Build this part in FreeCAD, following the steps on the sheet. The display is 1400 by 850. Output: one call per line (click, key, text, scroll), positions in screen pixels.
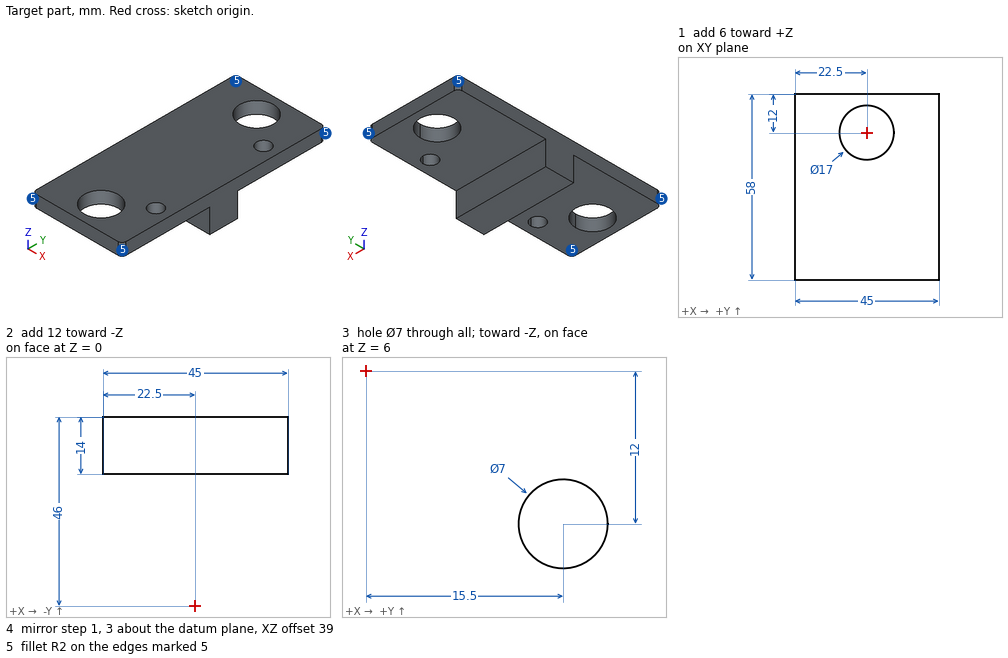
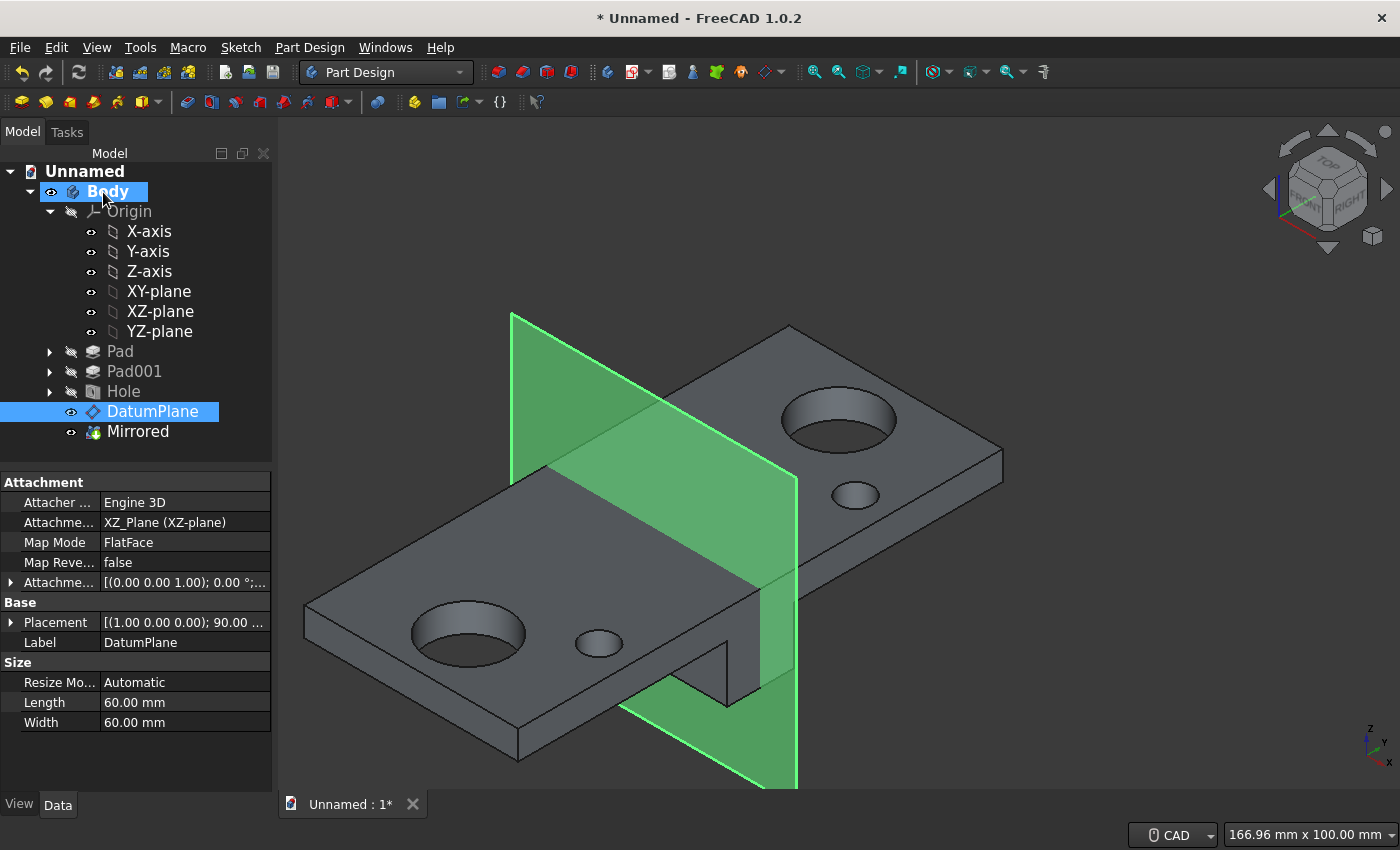
click(116, 412)
key(space)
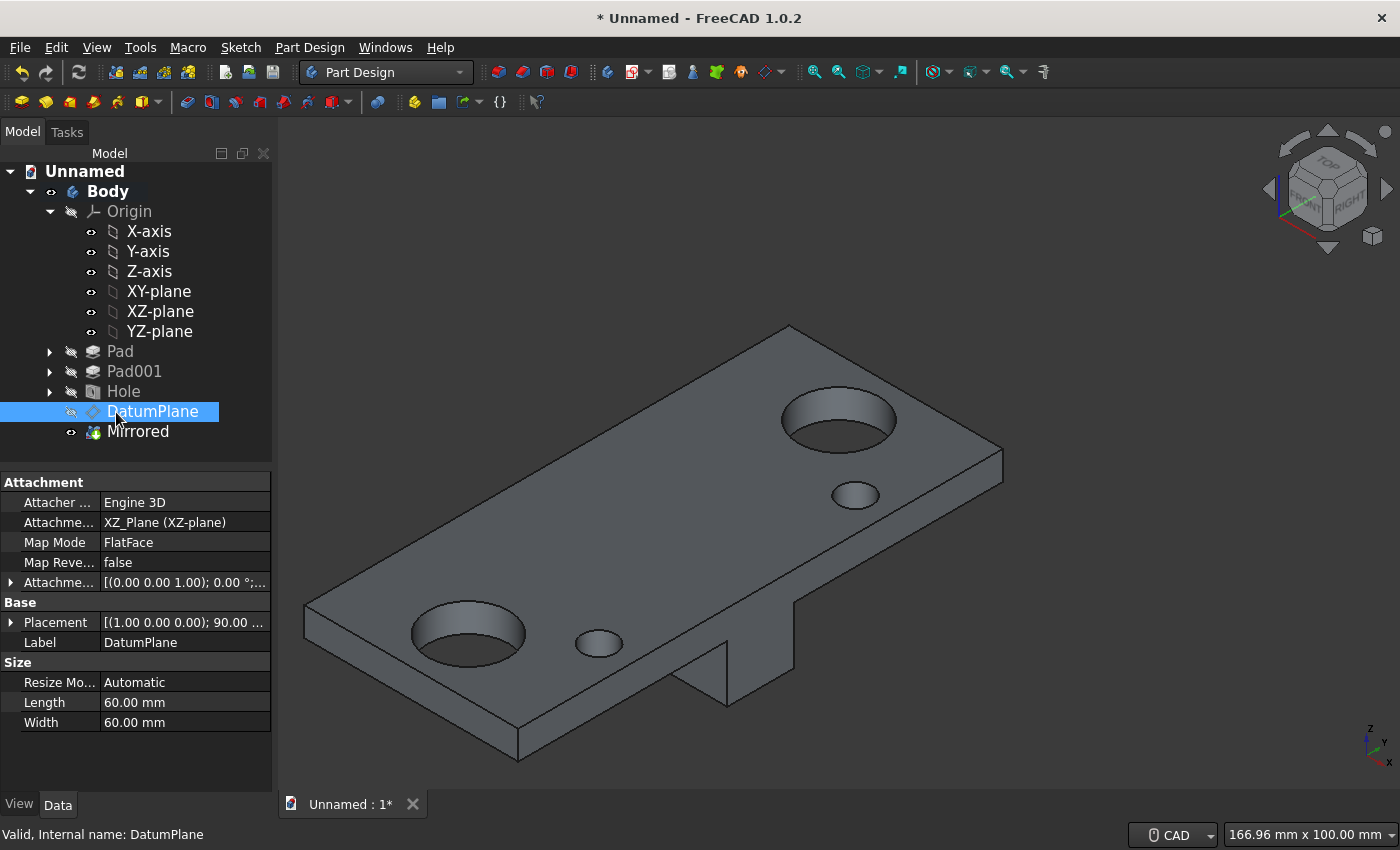
click(816, 72)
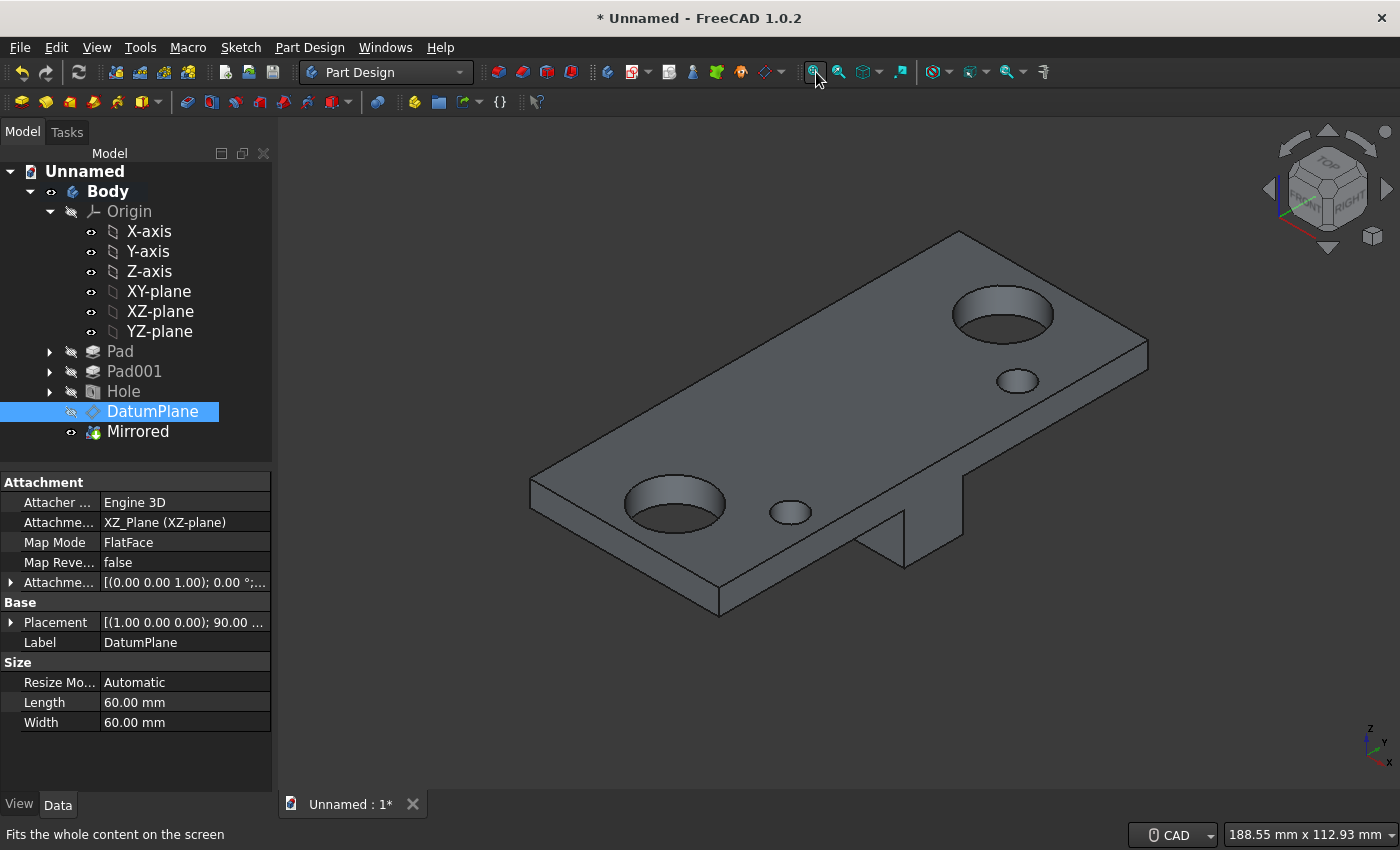
click(719, 601)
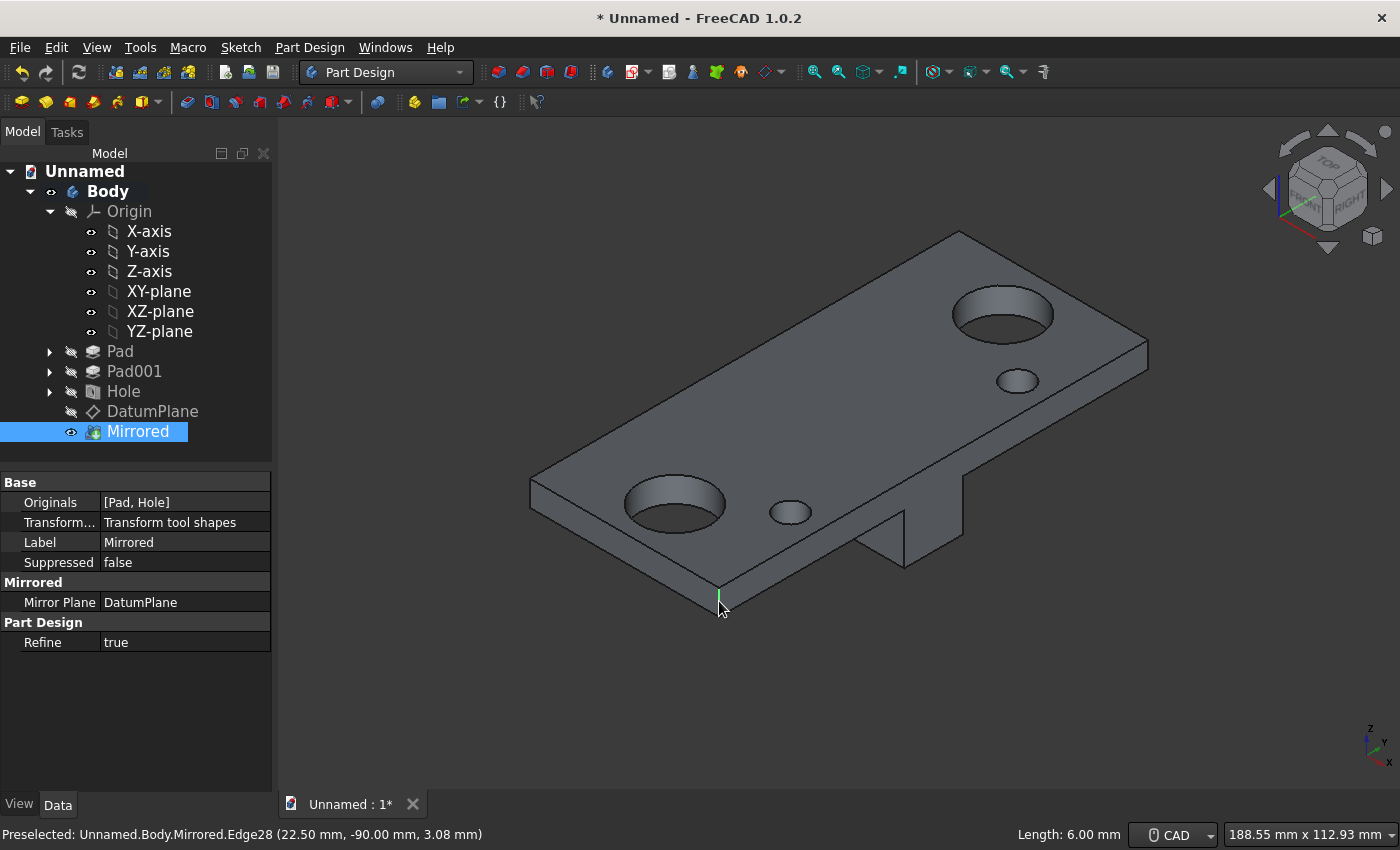
key(2)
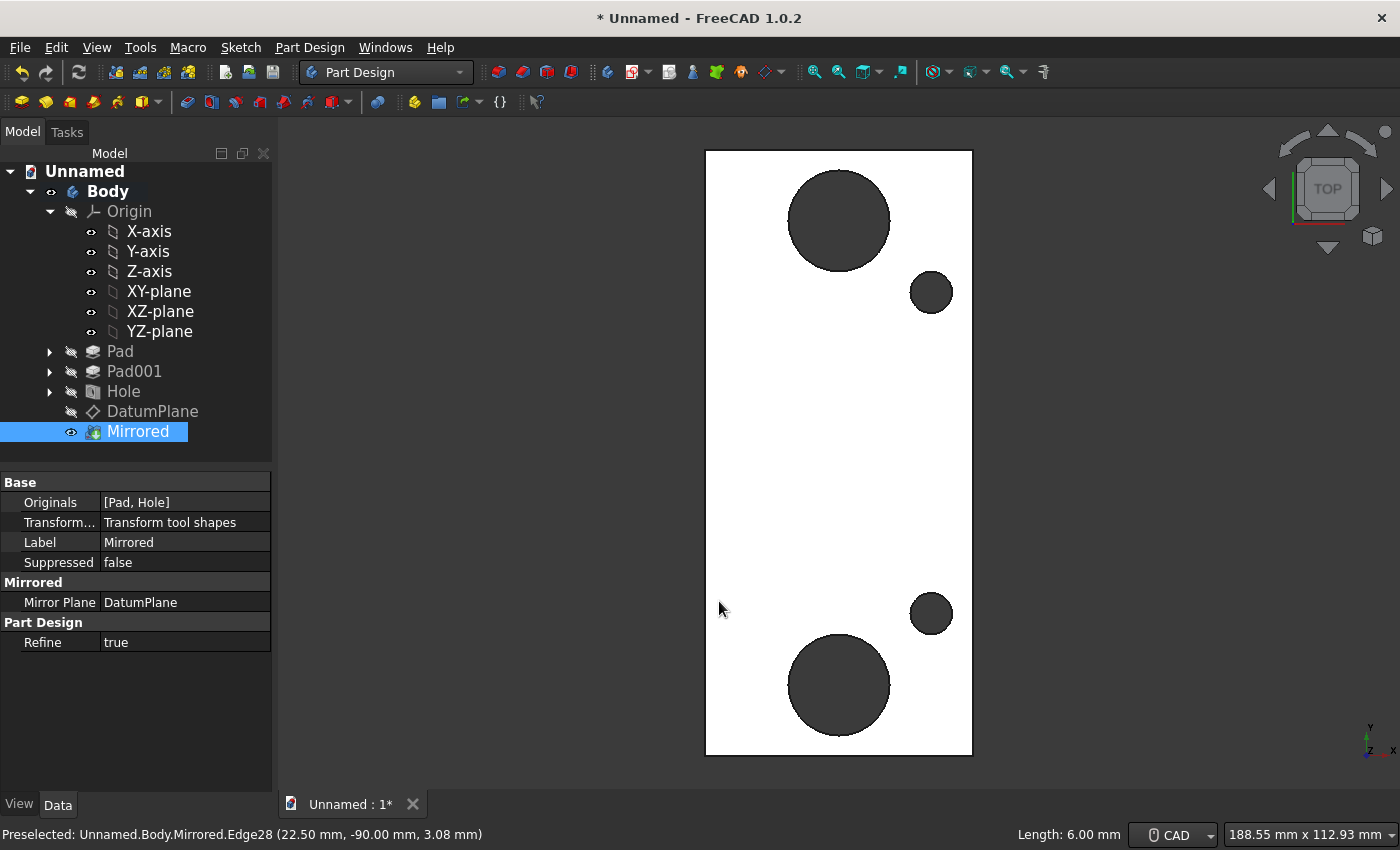
key(0)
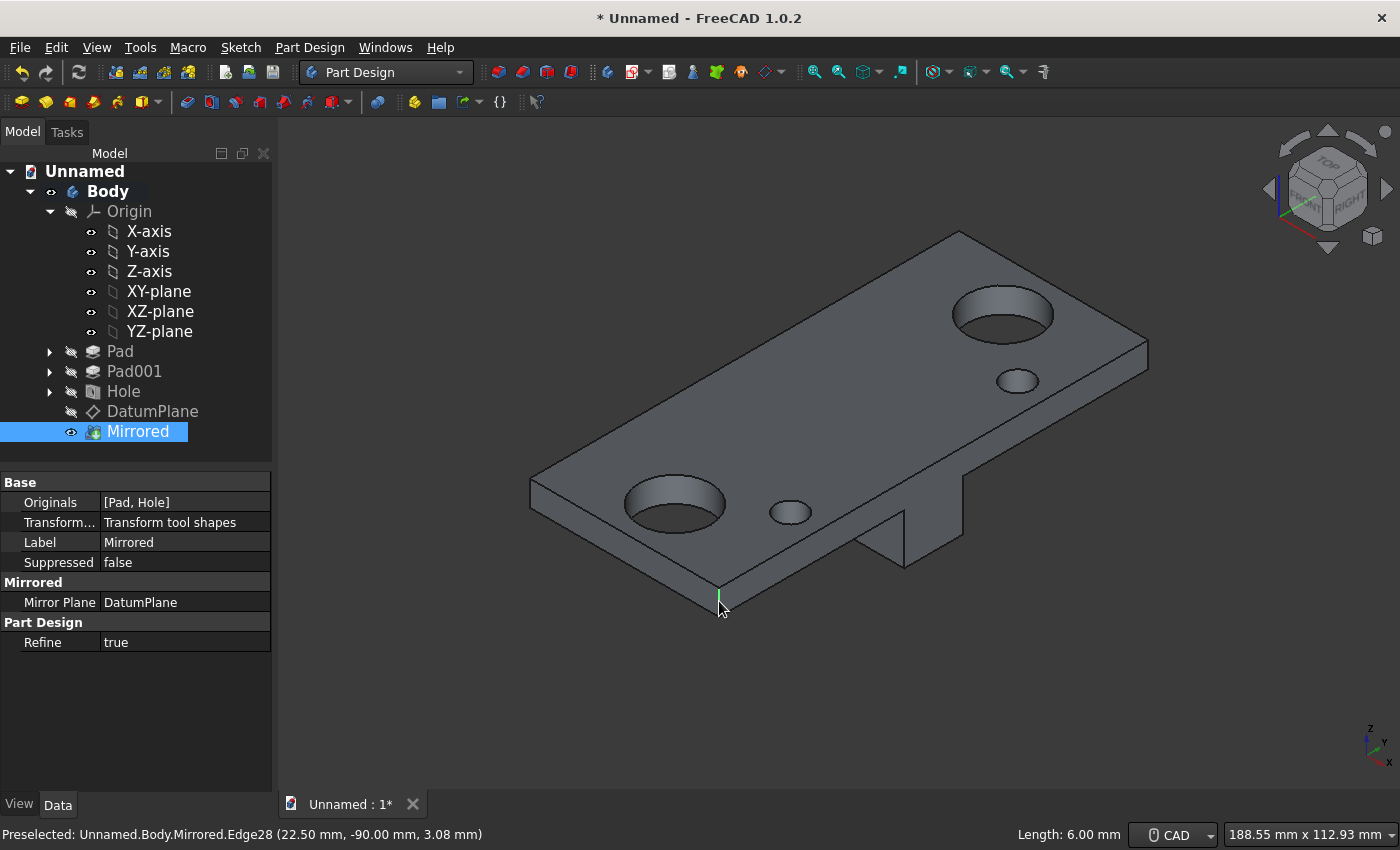
key(1)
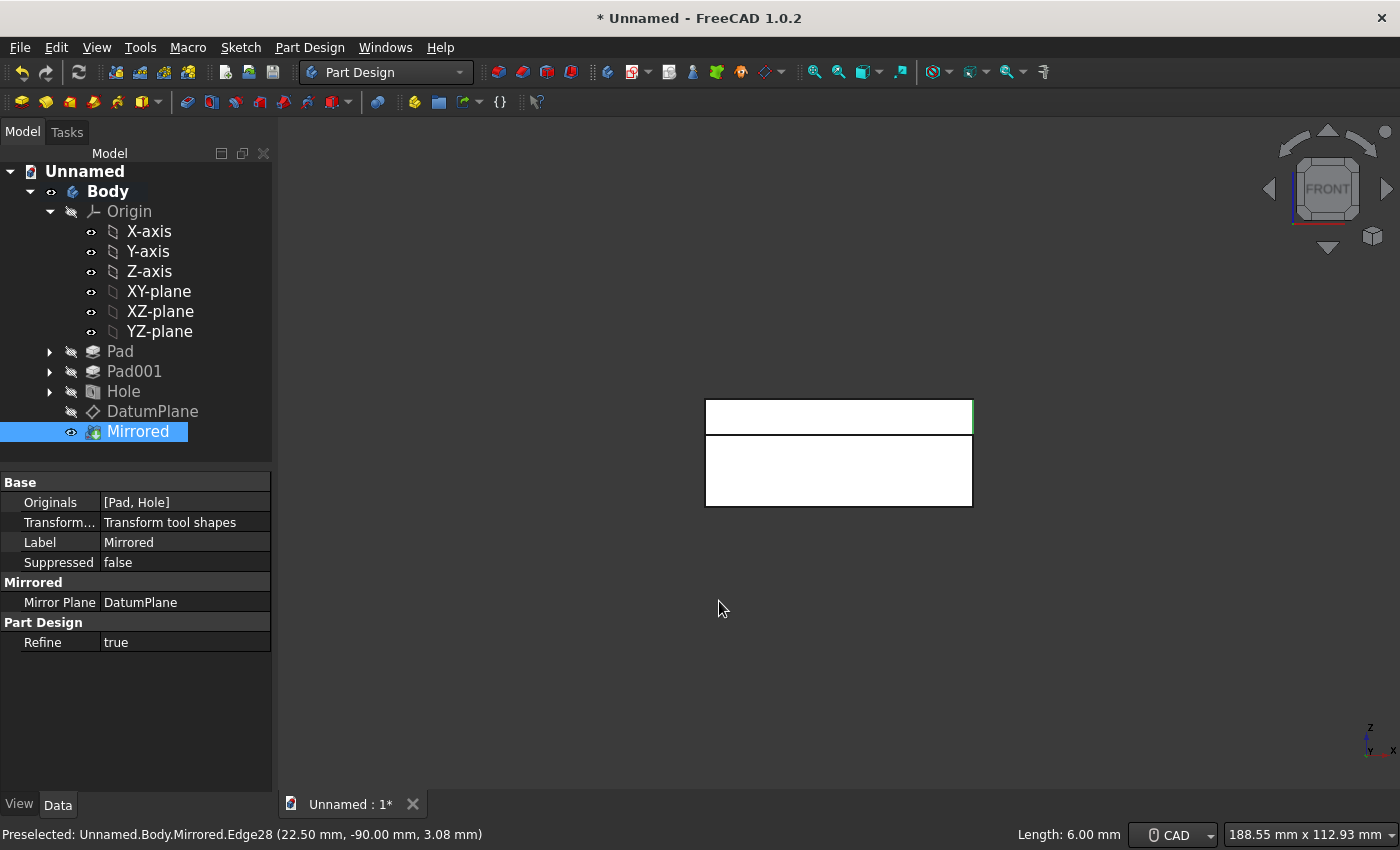
click(816, 72)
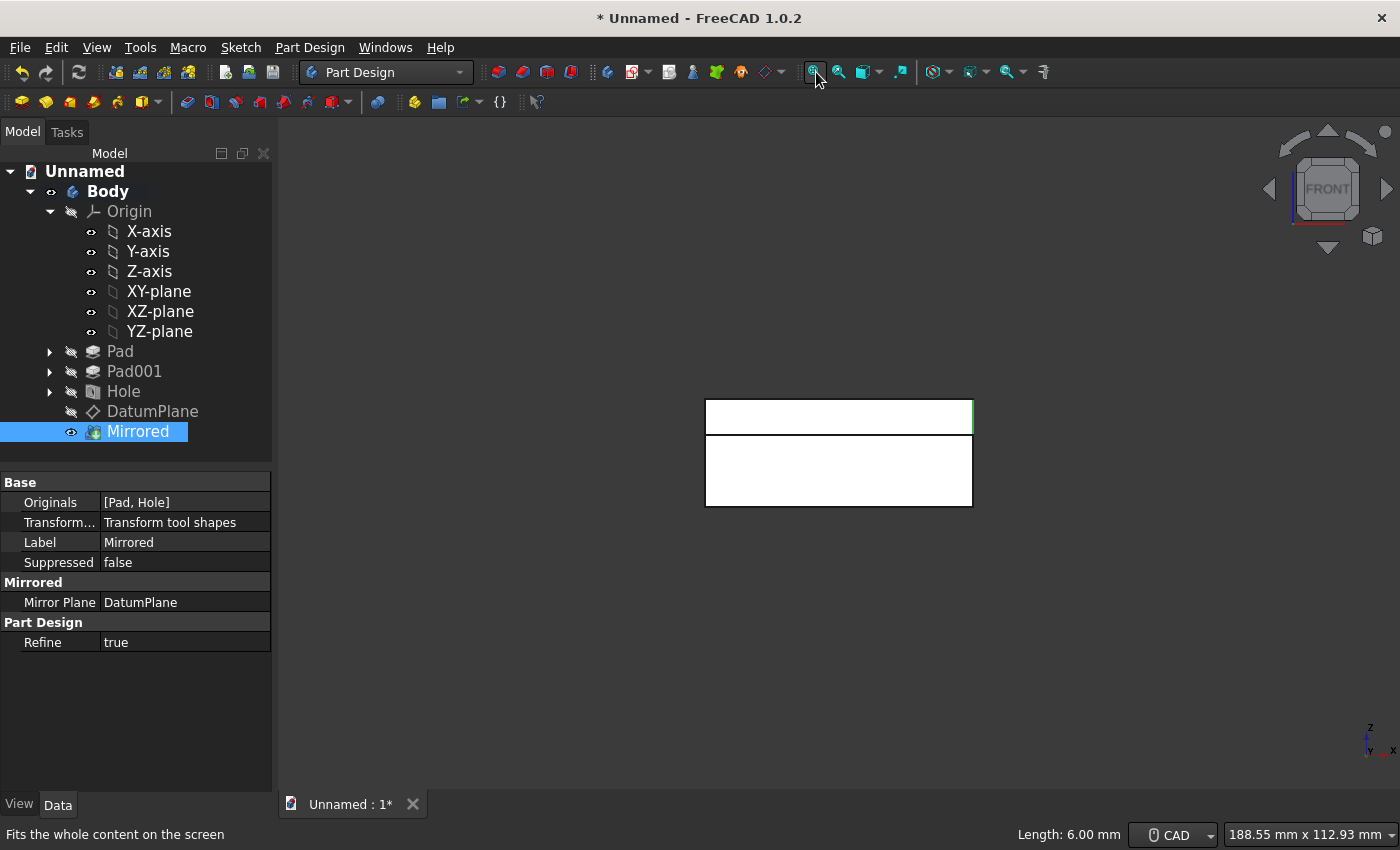
click(705, 416, ctrl)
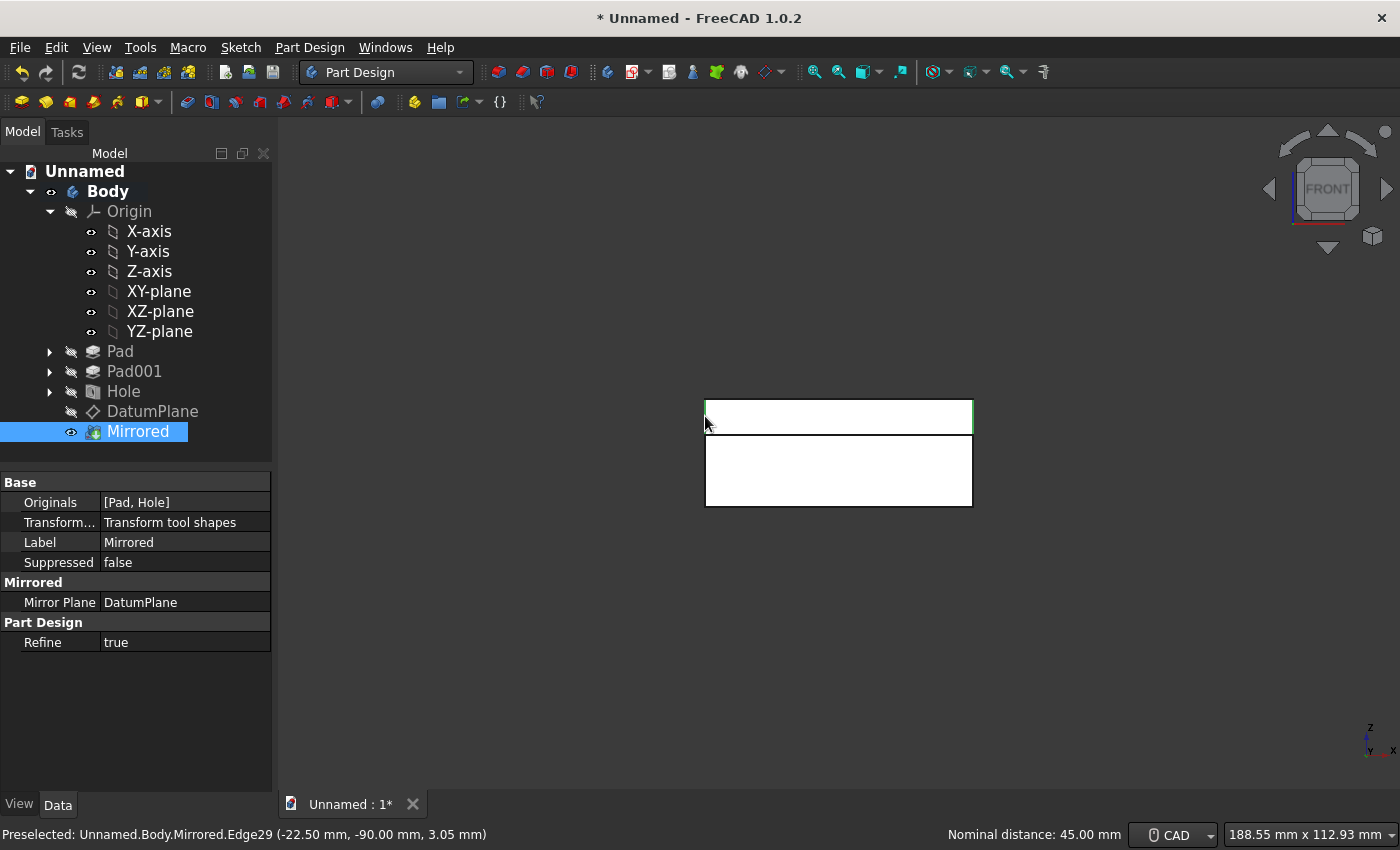
key(3)